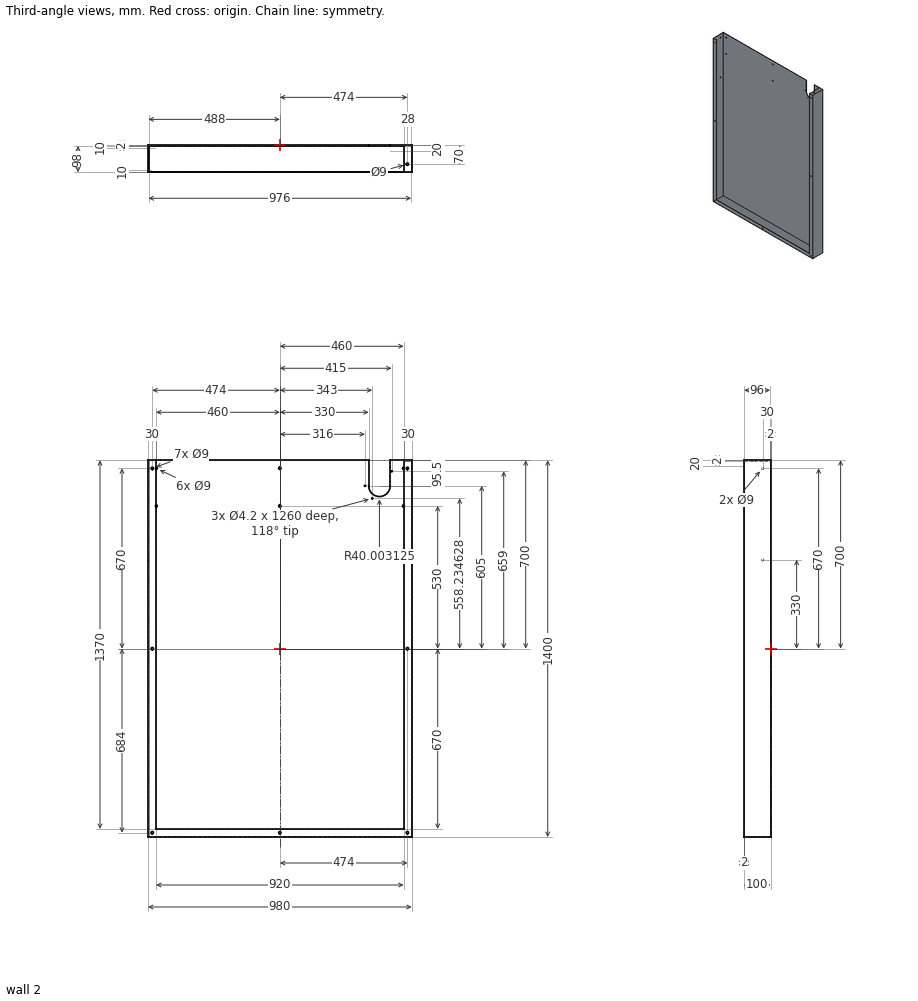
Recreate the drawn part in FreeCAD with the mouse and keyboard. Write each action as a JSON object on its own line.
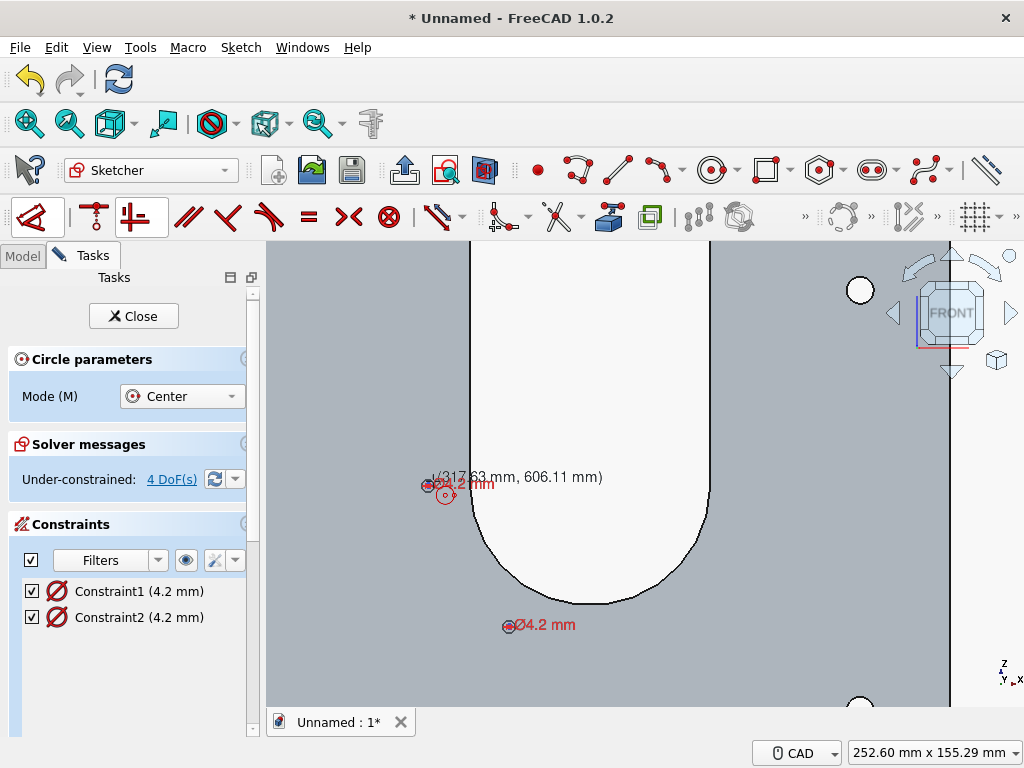
{"action": "scroll", "coordinate": [725, 323], "scroll_direction": "up", "scroll_amount": 7}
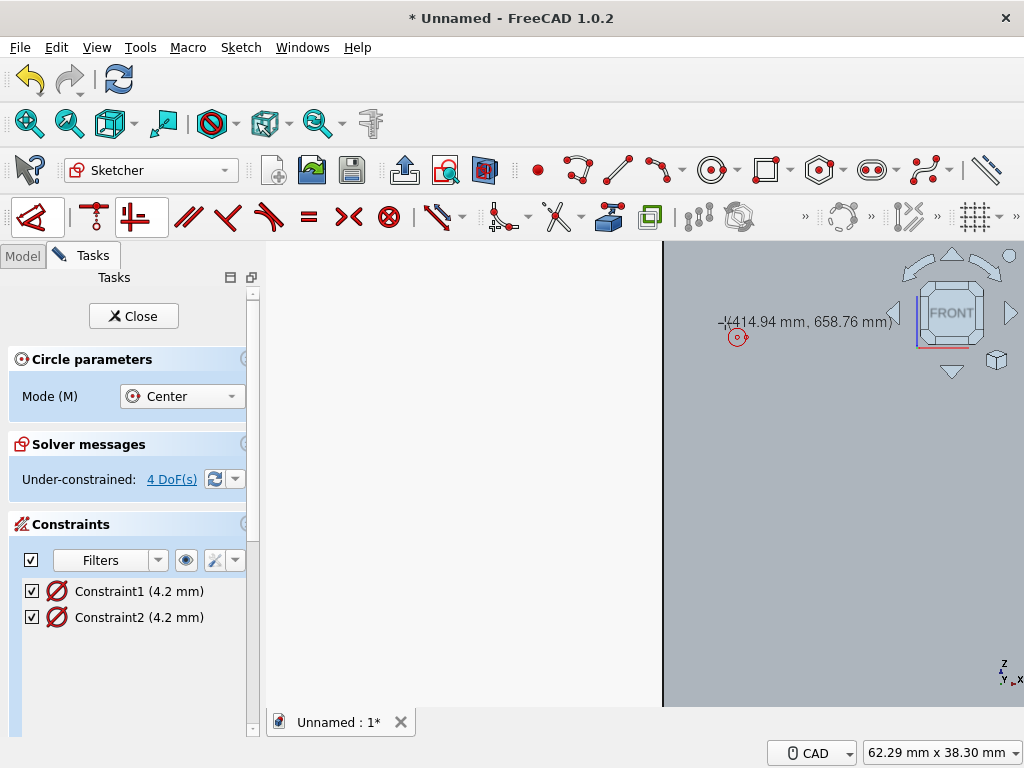
{"action": "scroll", "coordinate": [725, 323], "scroll_direction": "down", "scroll_amount": 7}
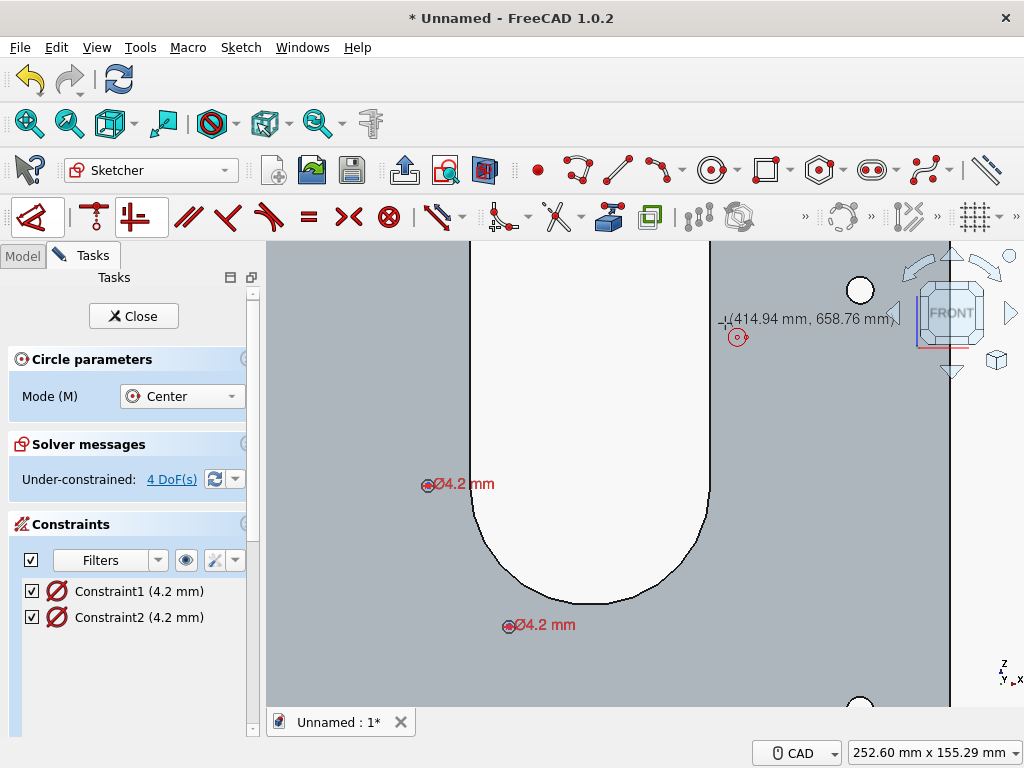
{"action": "left_click", "coordinate": [725, 323]}
{"action": "mouse_move", "coordinate": [730, 319]}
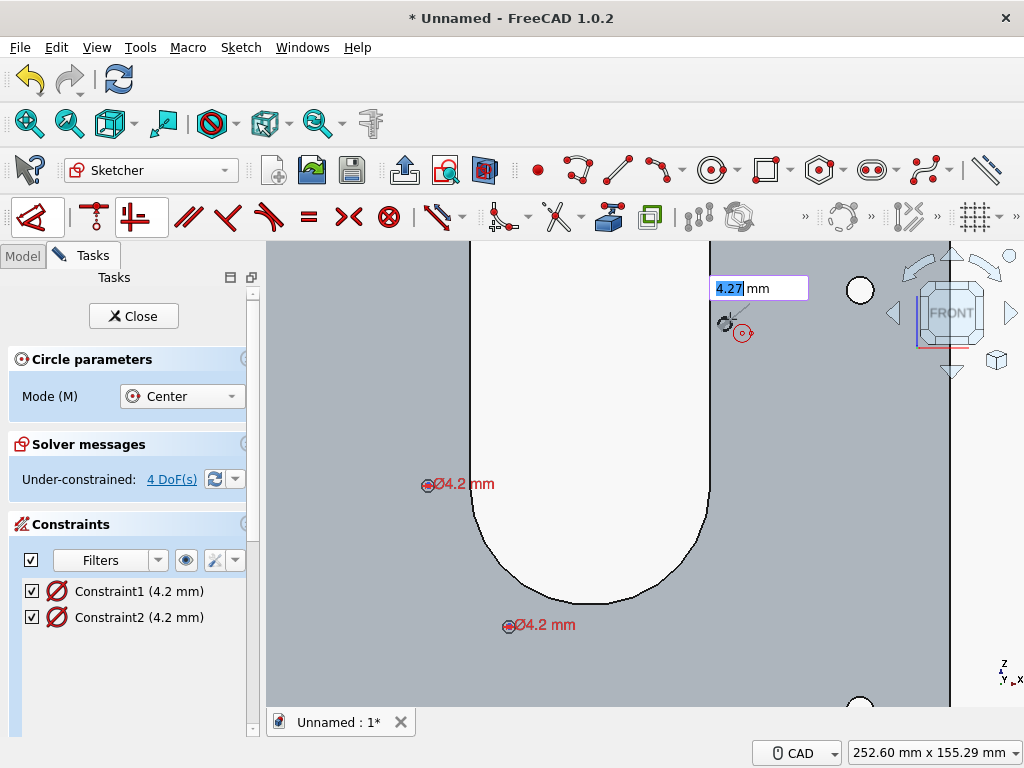
{"action": "type", "text": "4.2"}
{"action": "key", "text": "Return"}
{"action": "key", "text": "Escape"}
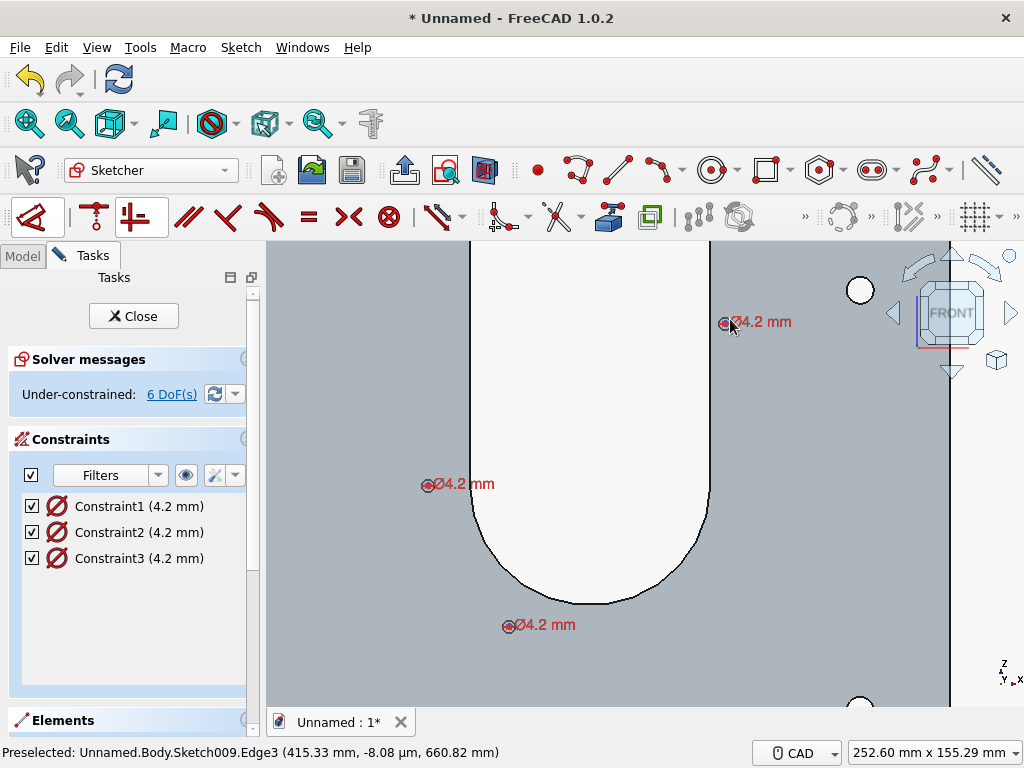
{"action": "left_click", "coordinate": [509, 627]}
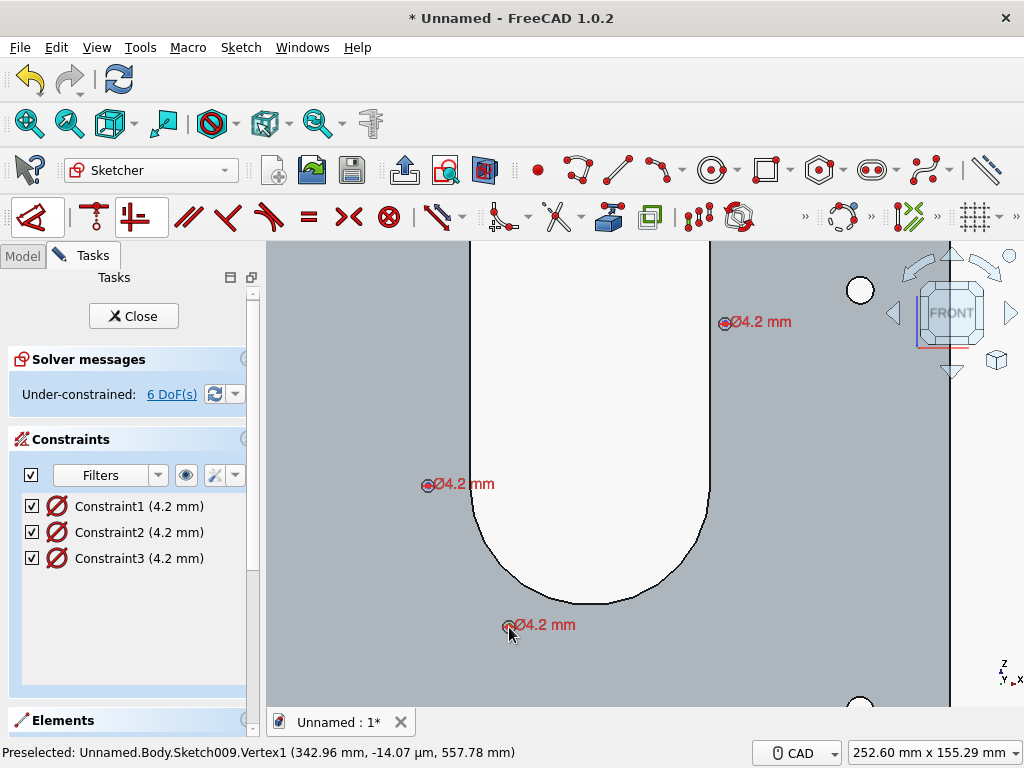
{"action": "left_click", "coordinate": [58, 218]}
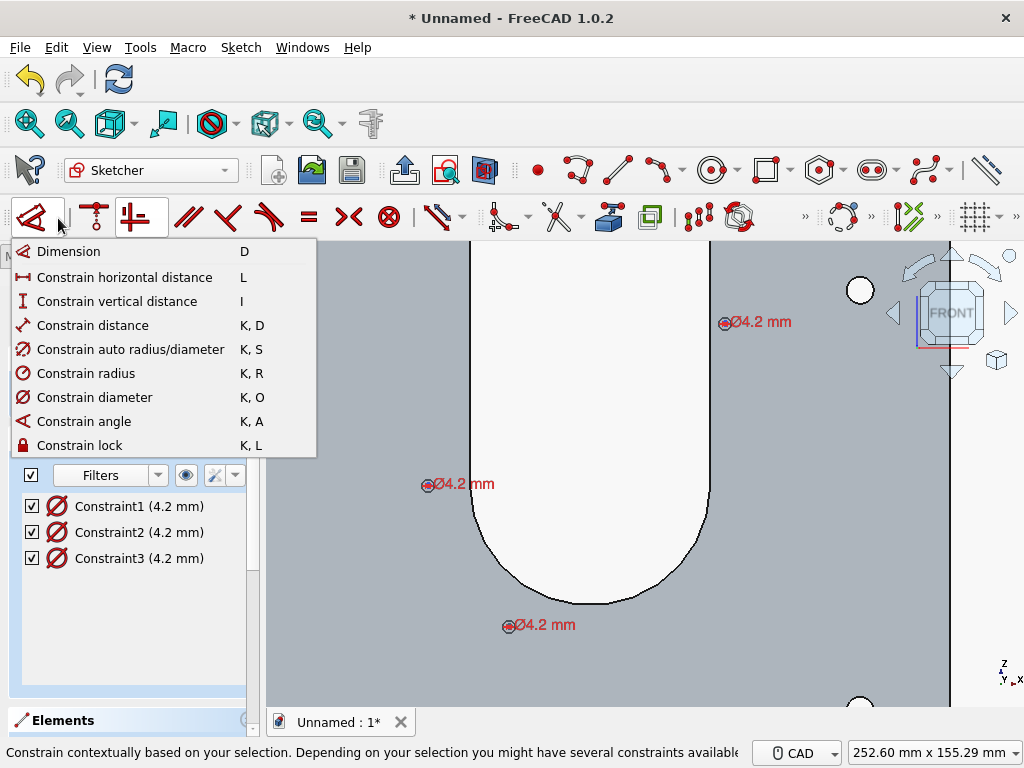
{"action": "left_click", "coordinate": [164, 277]}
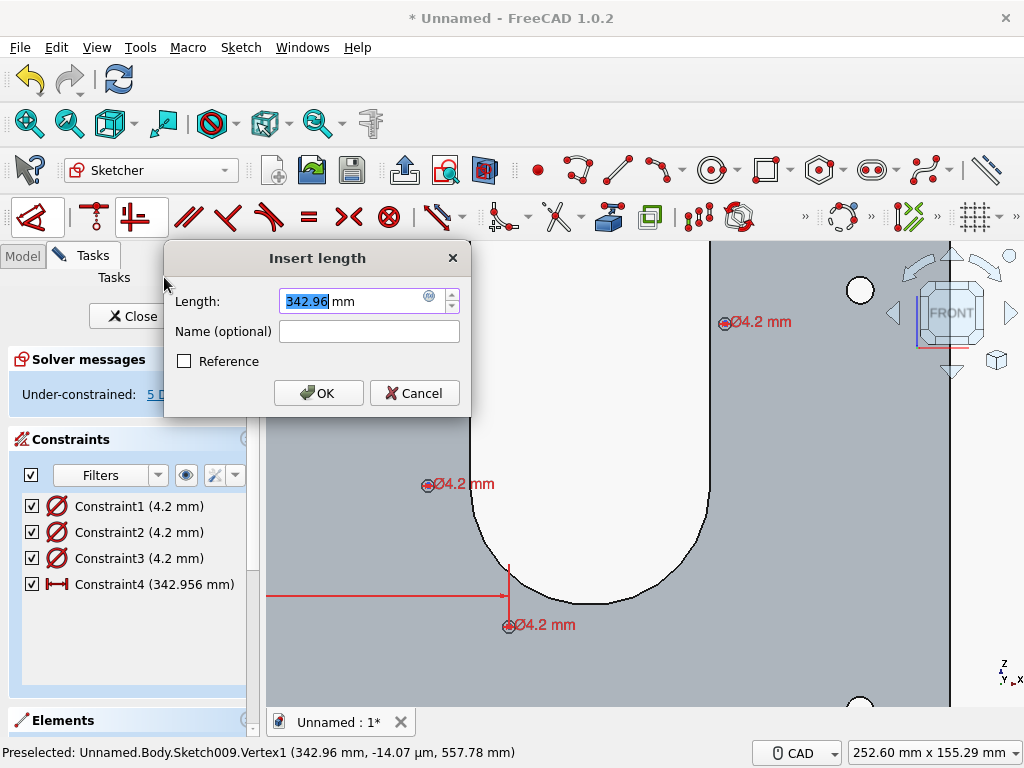
{"action": "type", "text": "343"}
{"action": "key", "text": "Return"}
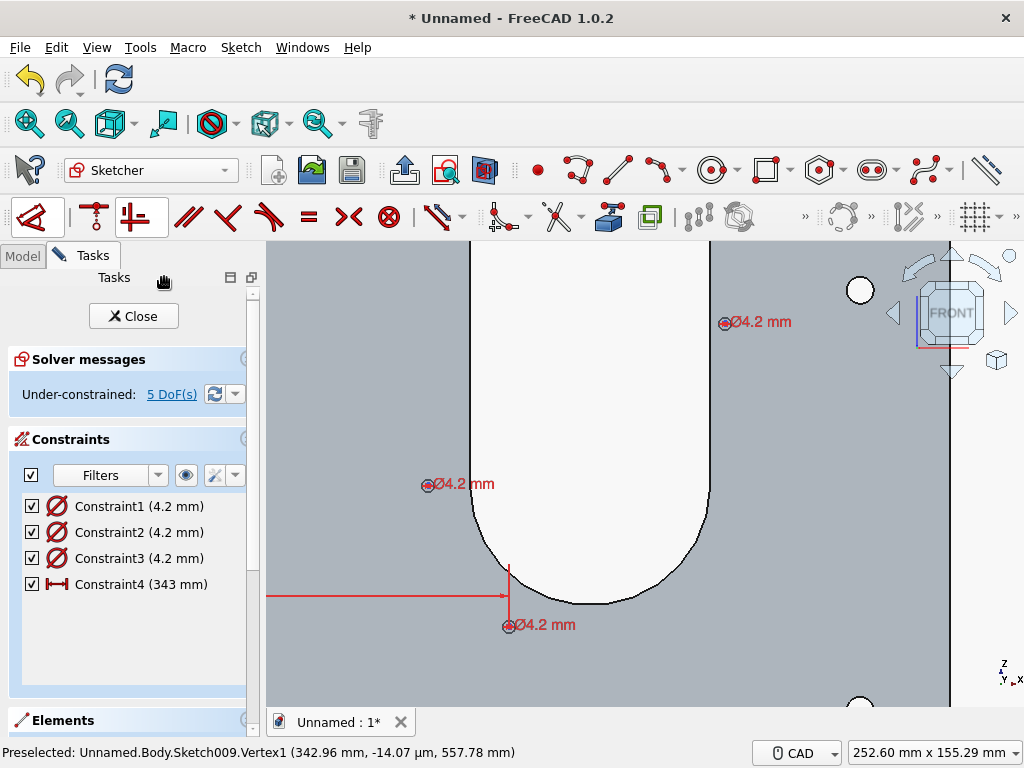
{"action": "left_click", "coordinate": [428, 486]}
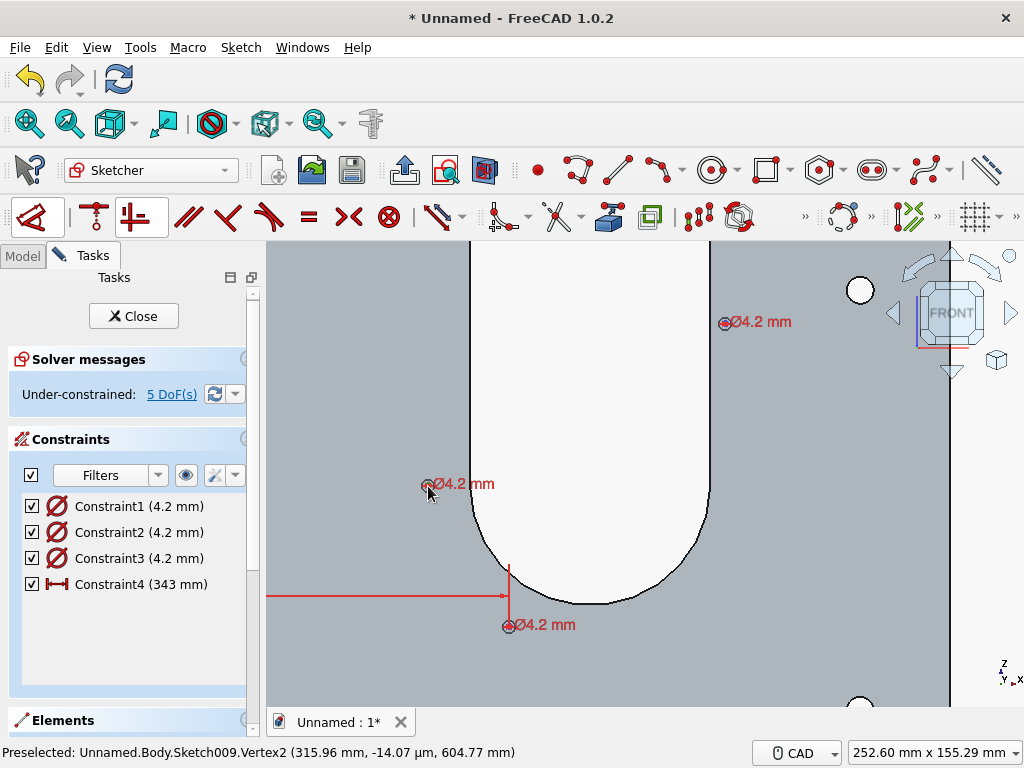
{"action": "left_click", "coordinate": [58, 218]}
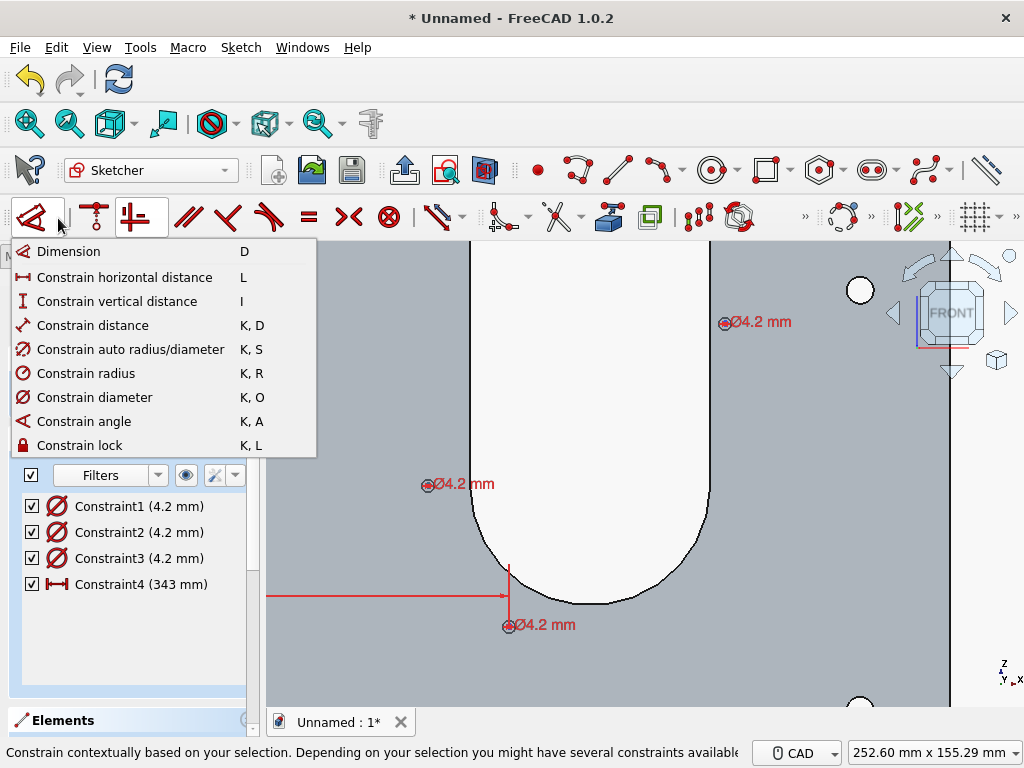
{"action": "left_click", "coordinate": [164, 277]}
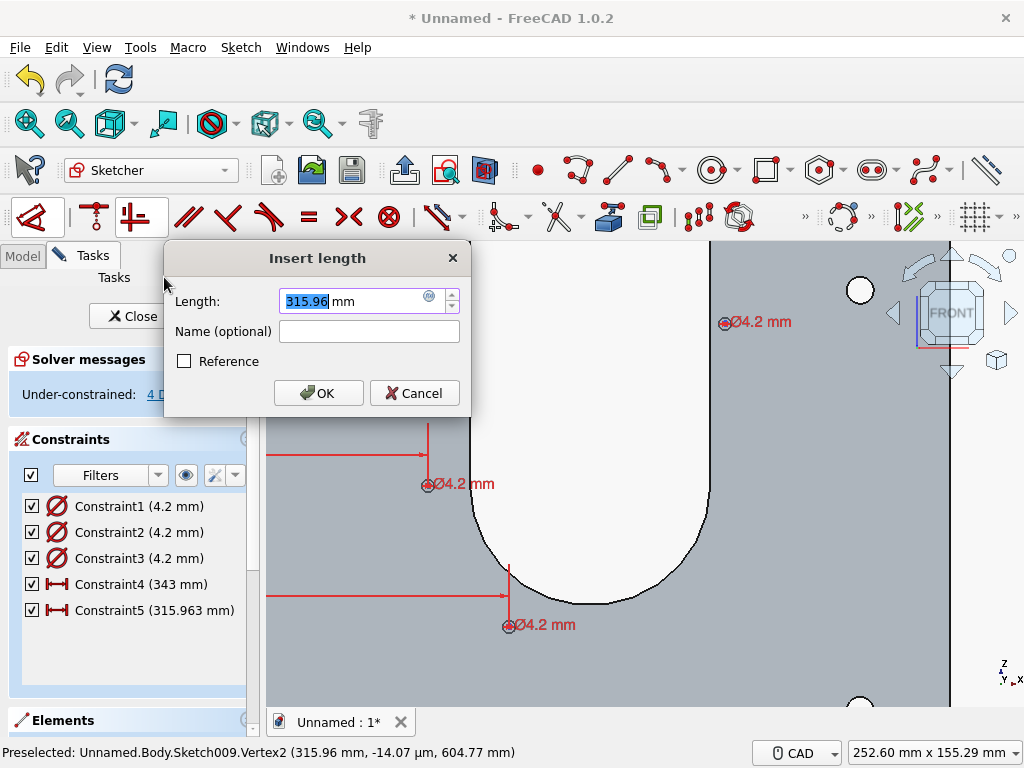
{"action": "type", "text": "316"}
{"action": "key", "text": "Return"}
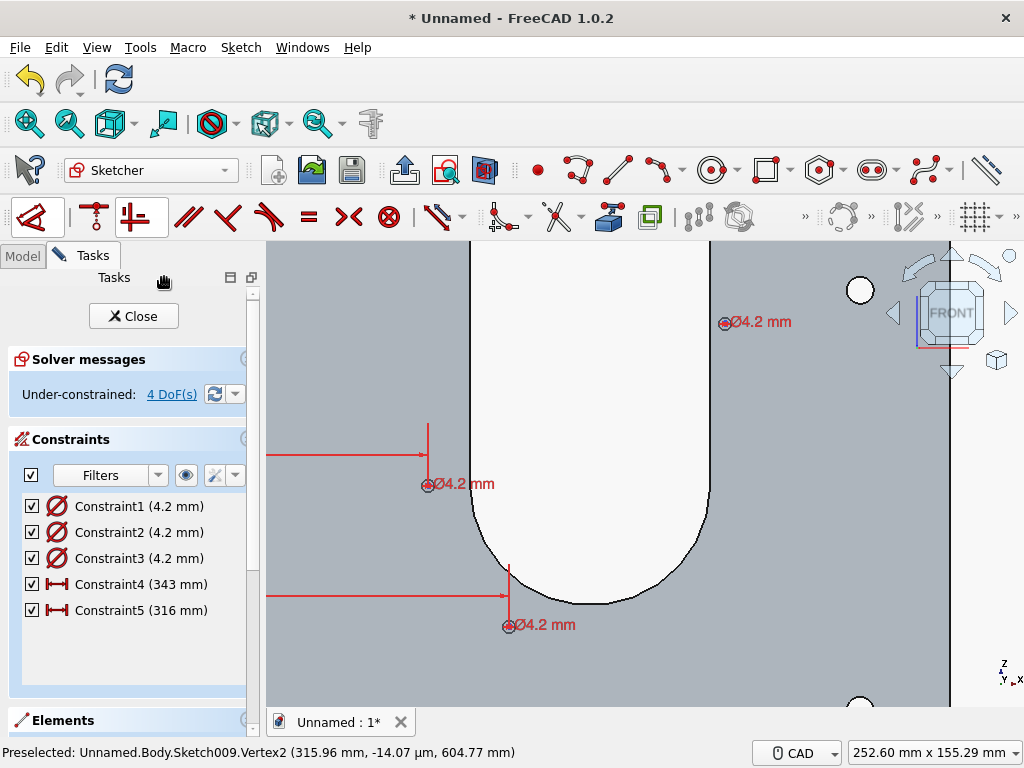
{"action": "left_click", "coordinate": [428, 486]}